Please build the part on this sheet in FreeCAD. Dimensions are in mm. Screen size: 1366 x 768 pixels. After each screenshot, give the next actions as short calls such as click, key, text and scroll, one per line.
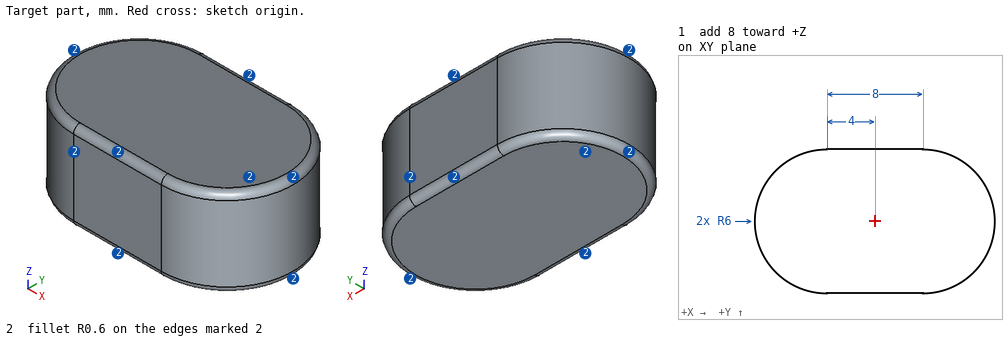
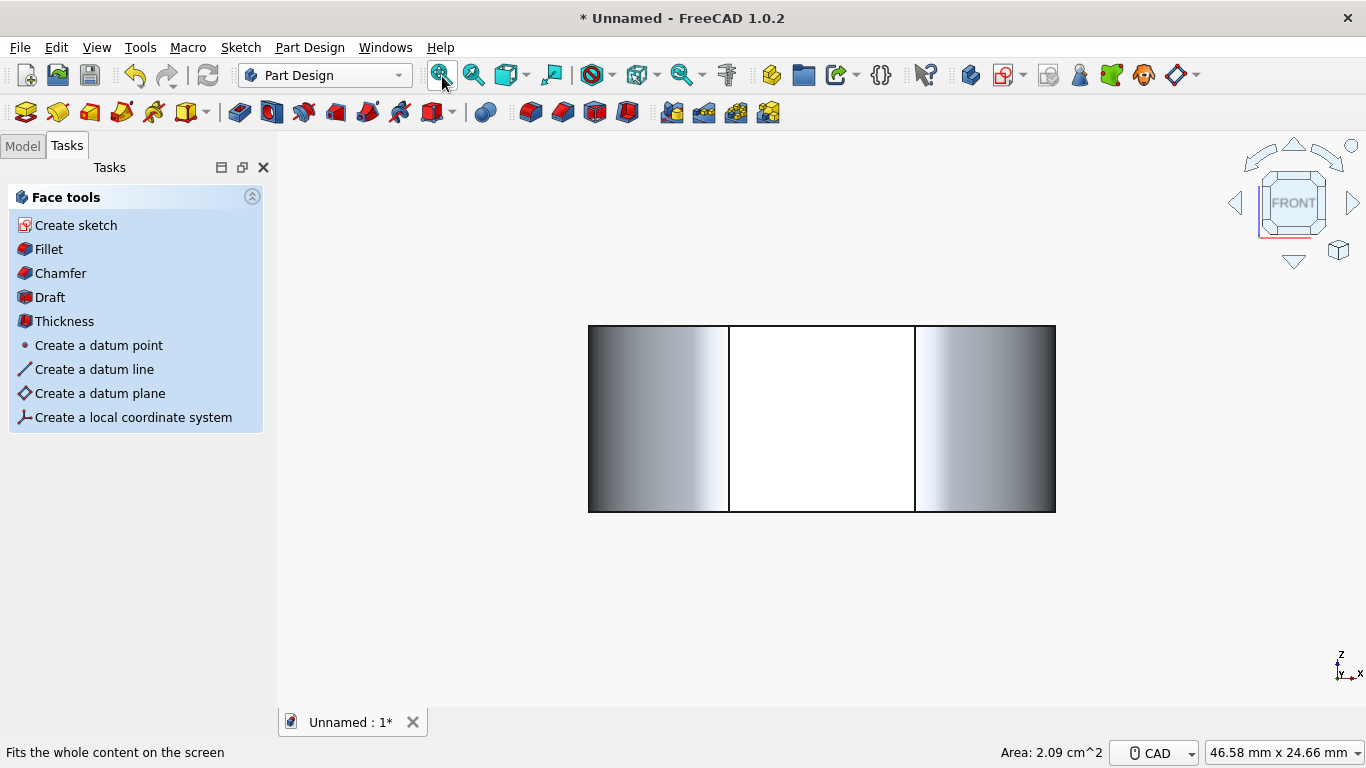
key(3)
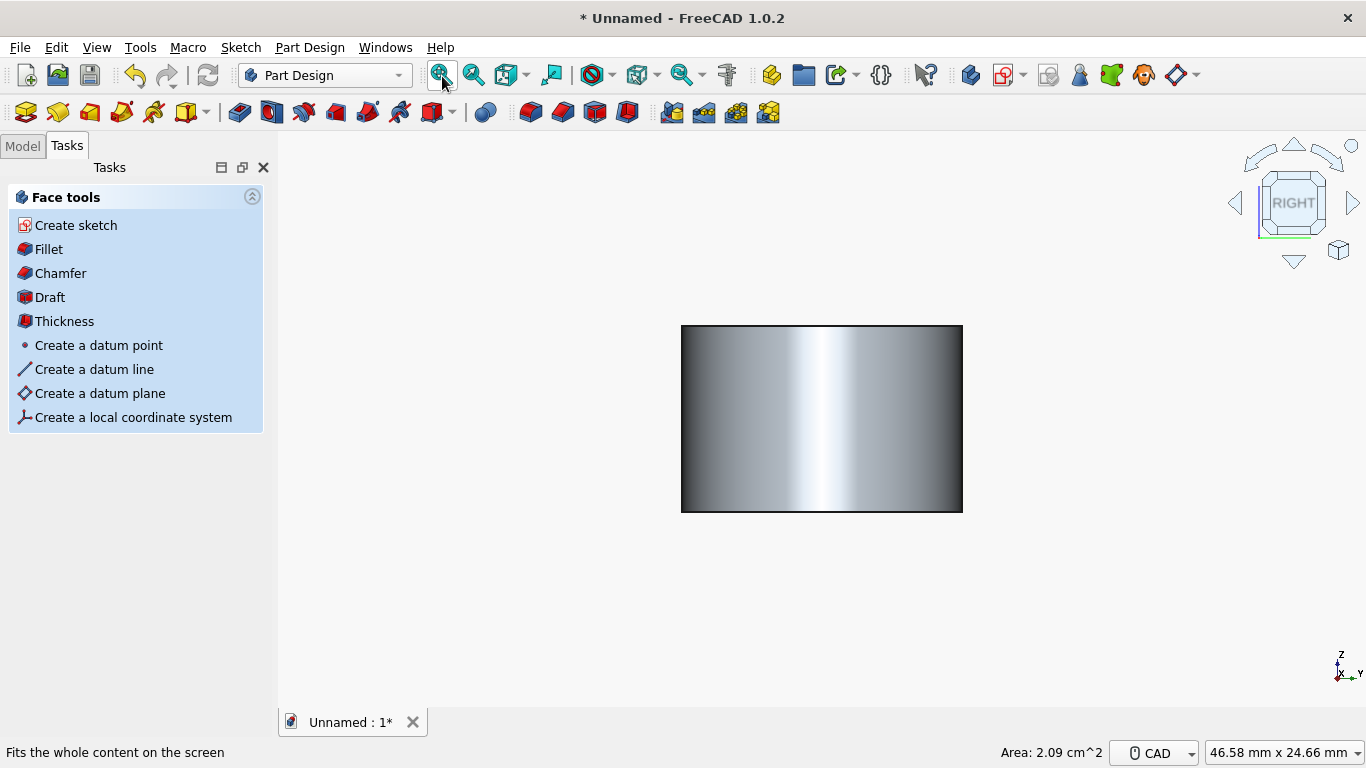
click(442, 76)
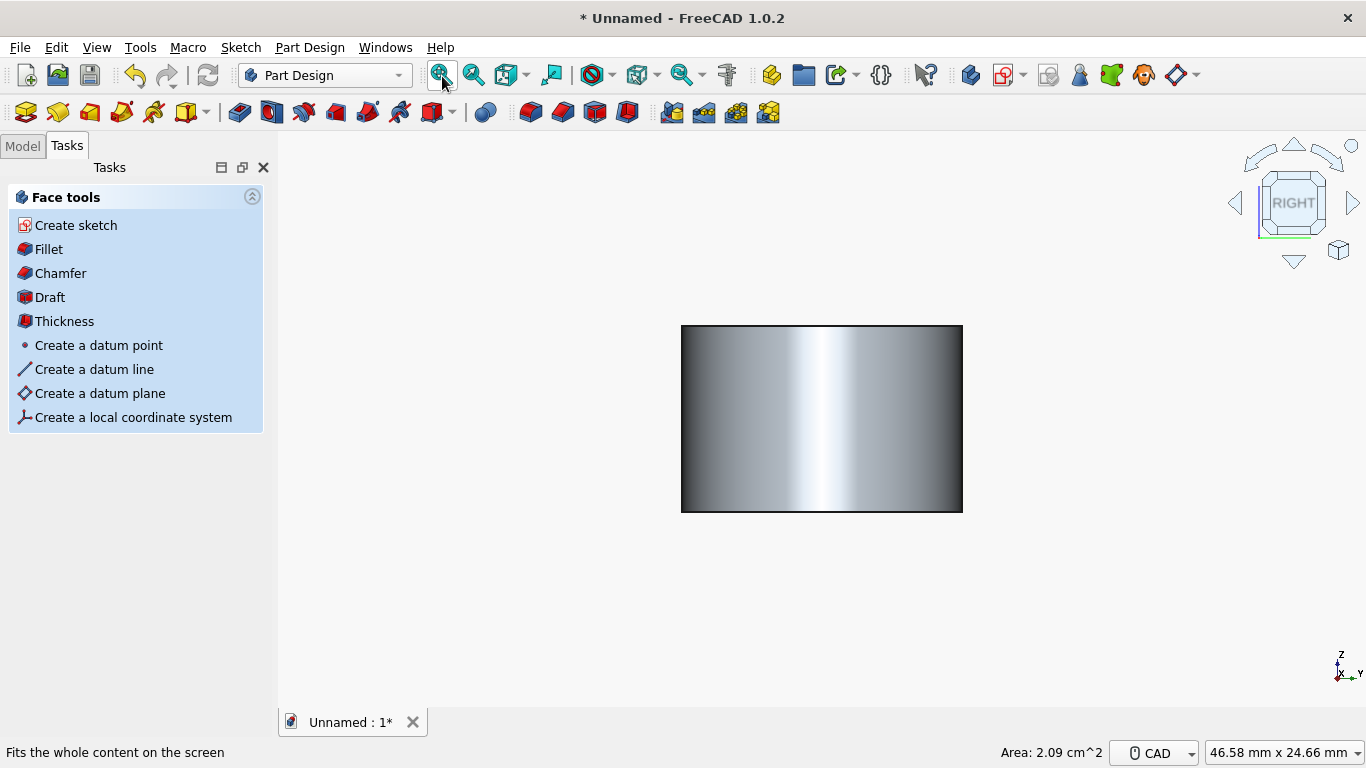
key(5)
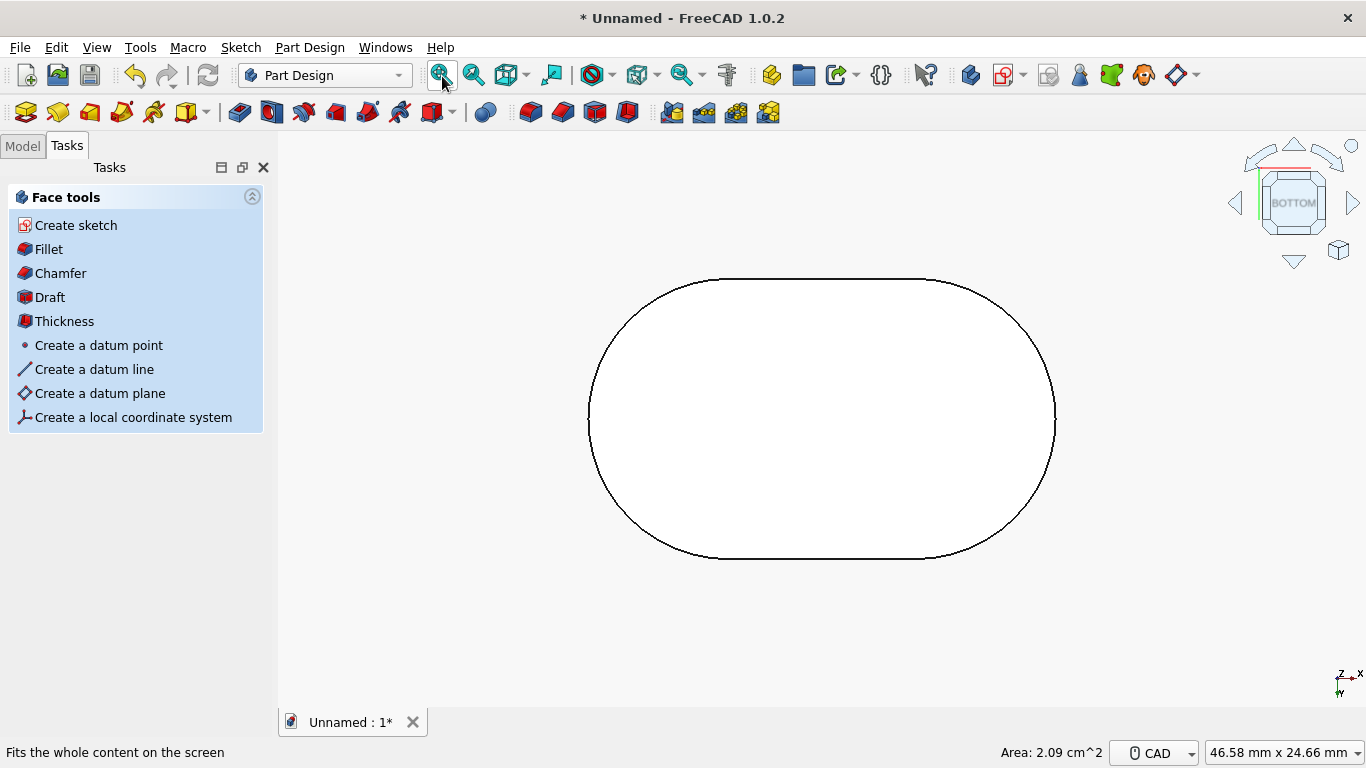
click(889, 418, ctrl)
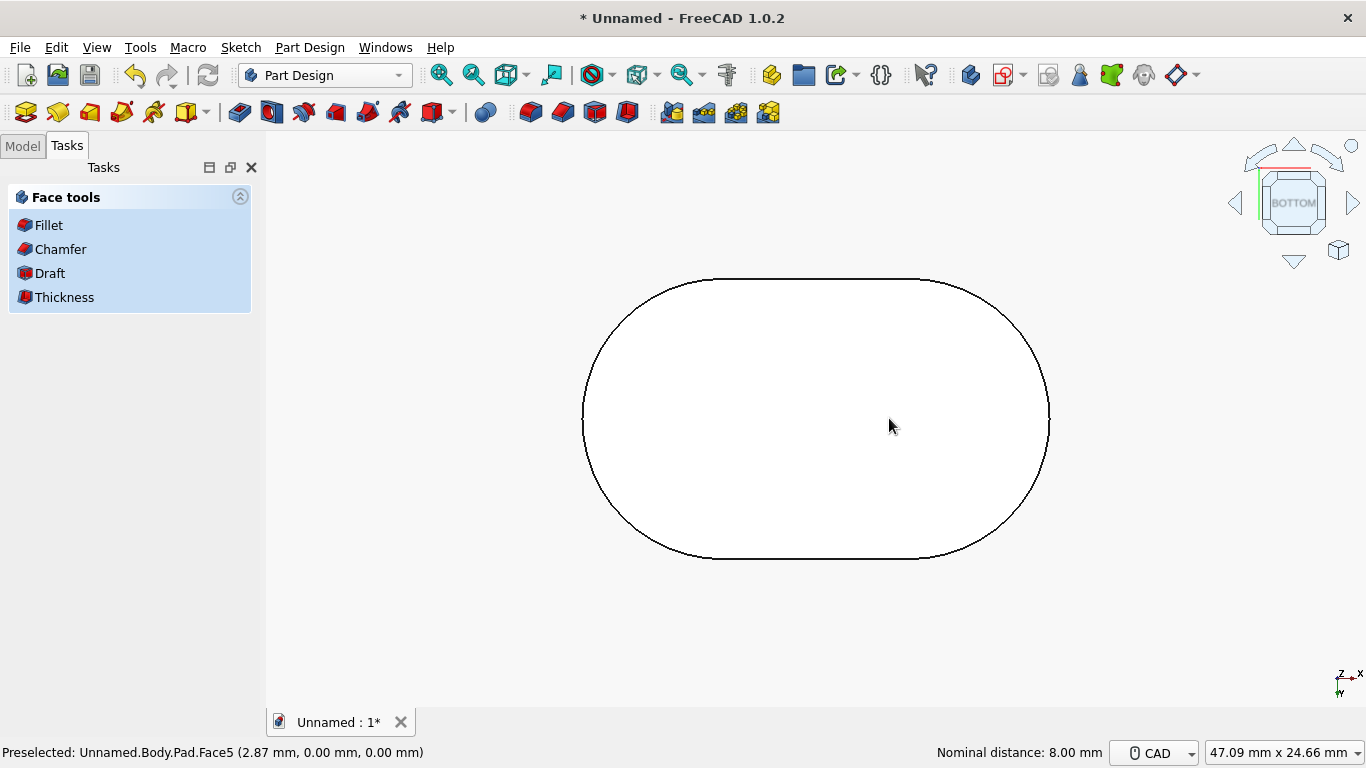
click(532, 112)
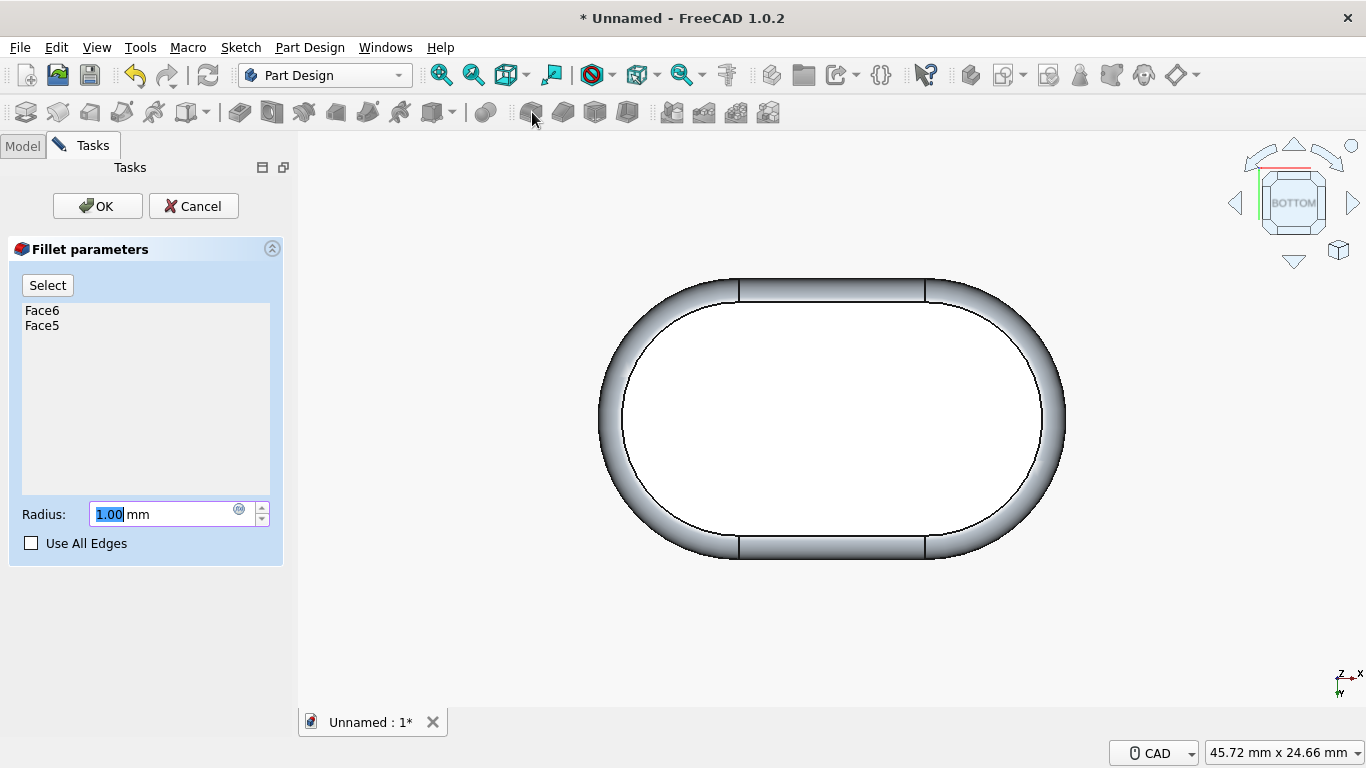
text(0.6)
key(Tab)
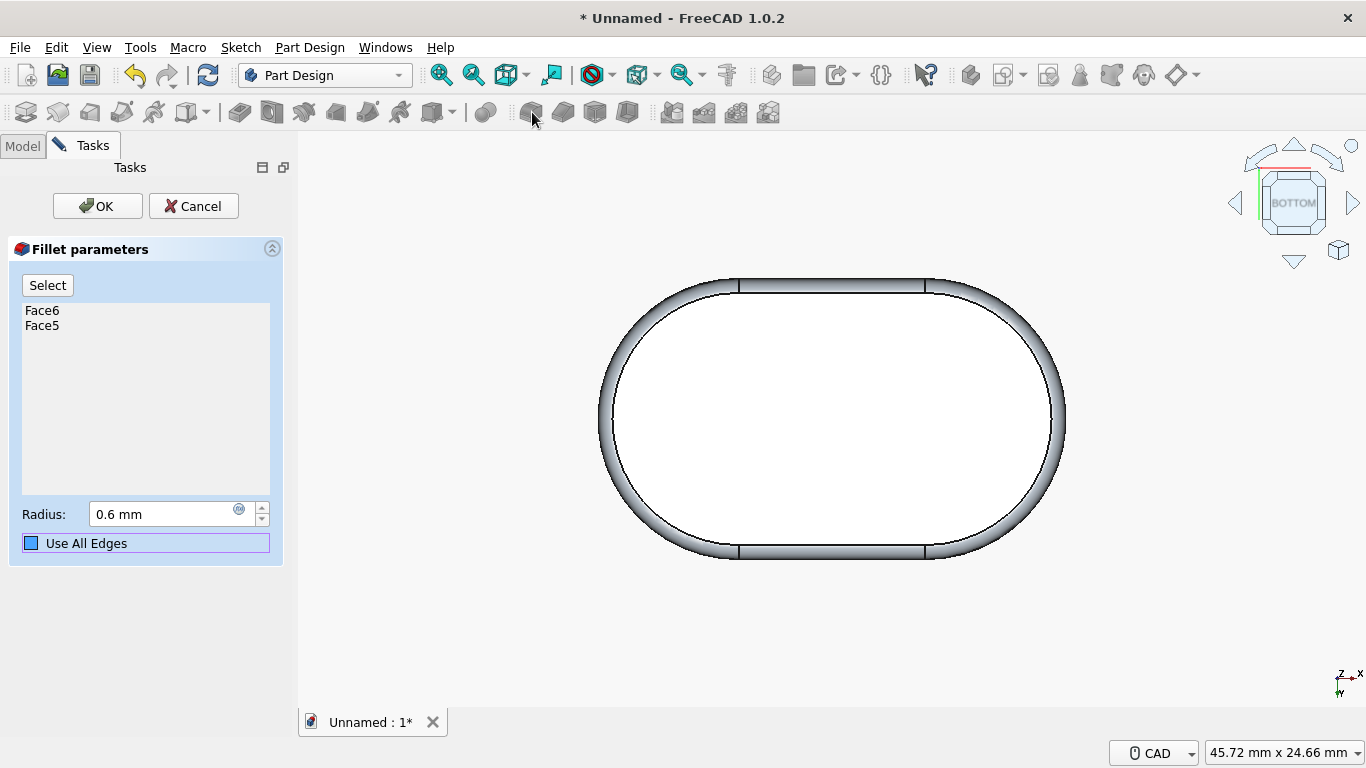
click(98, 206)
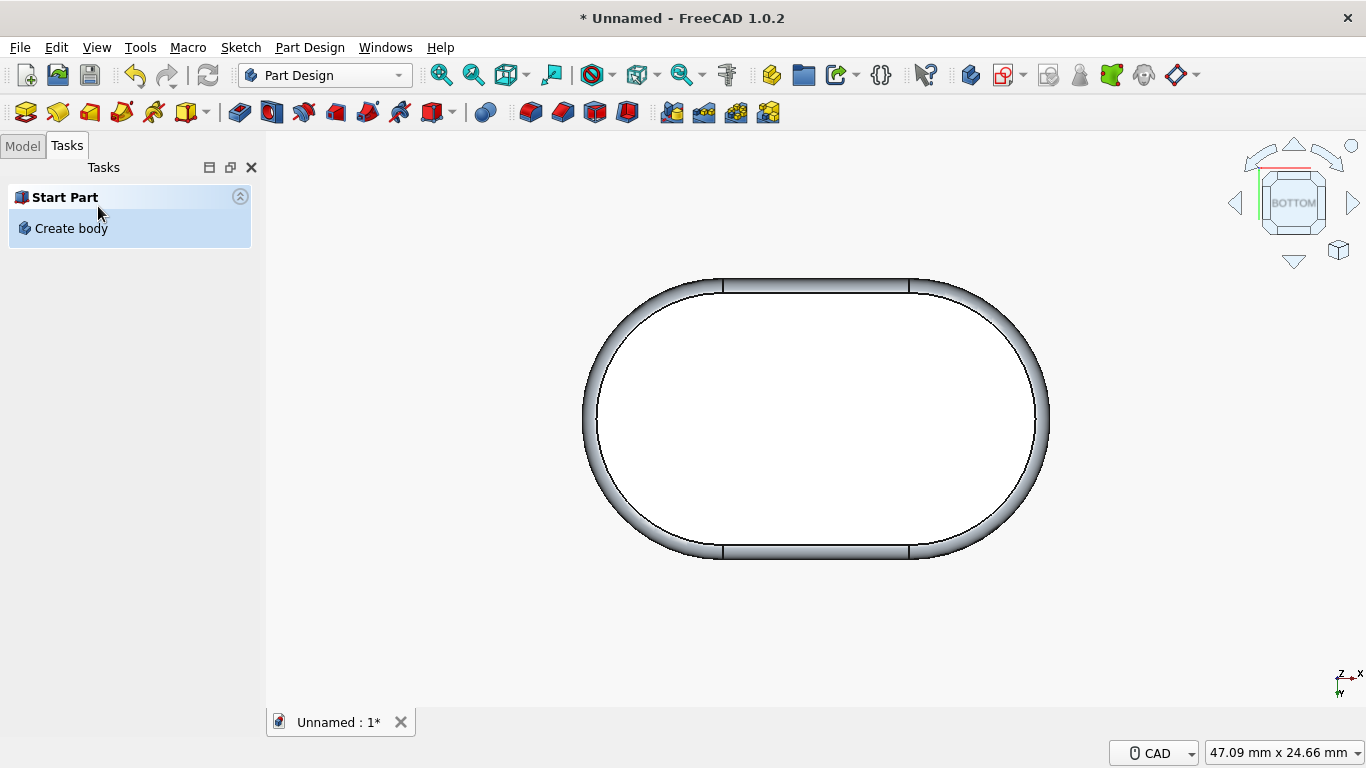
key(0)